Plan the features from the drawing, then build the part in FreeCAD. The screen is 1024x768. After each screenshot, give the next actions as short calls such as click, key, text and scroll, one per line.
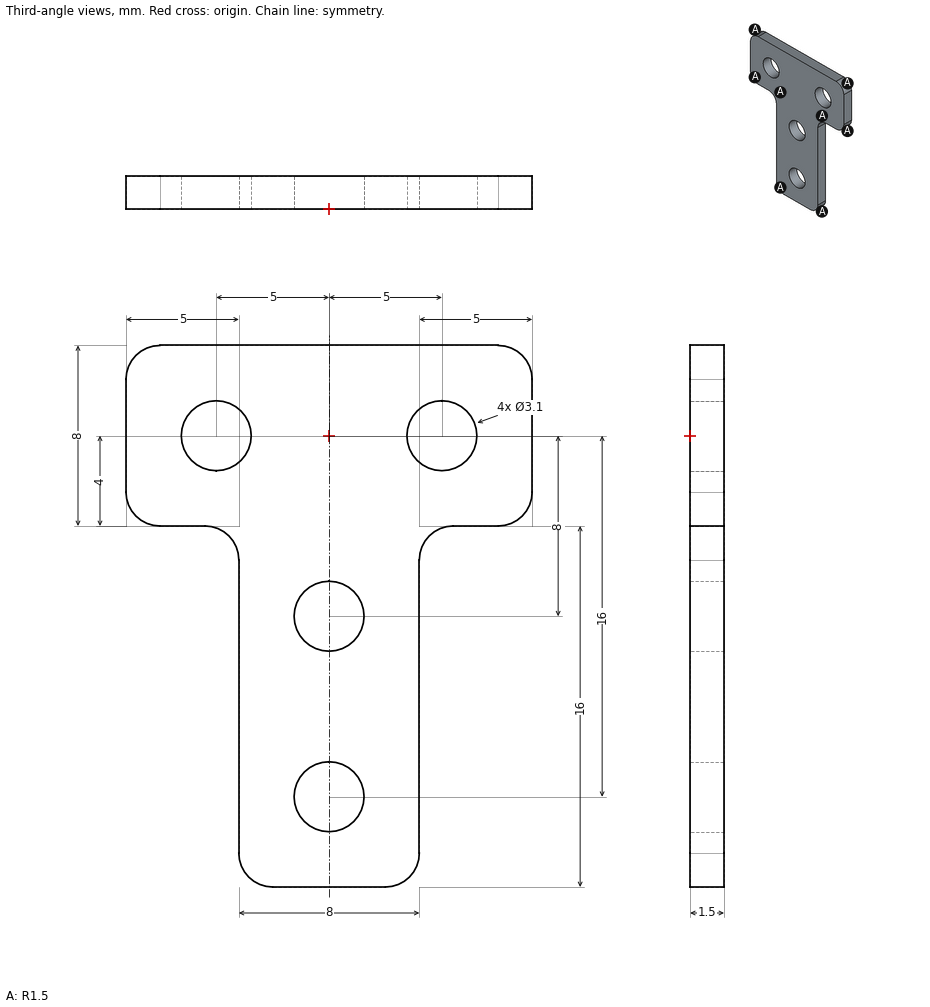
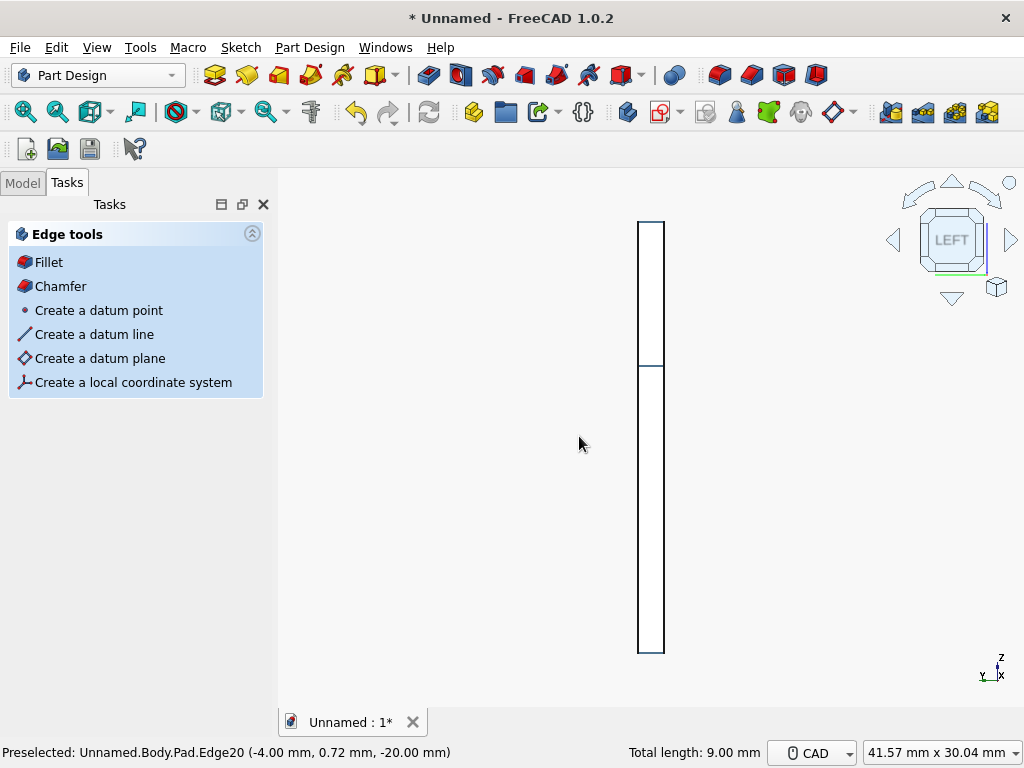
key(v)
key(3)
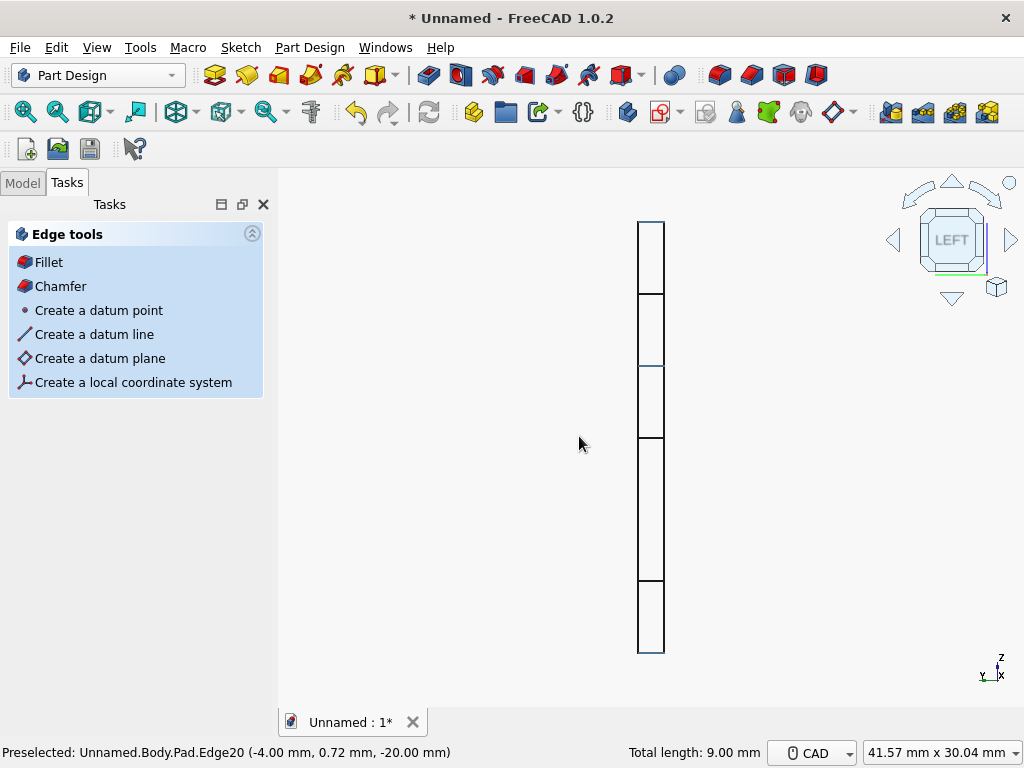
key(0)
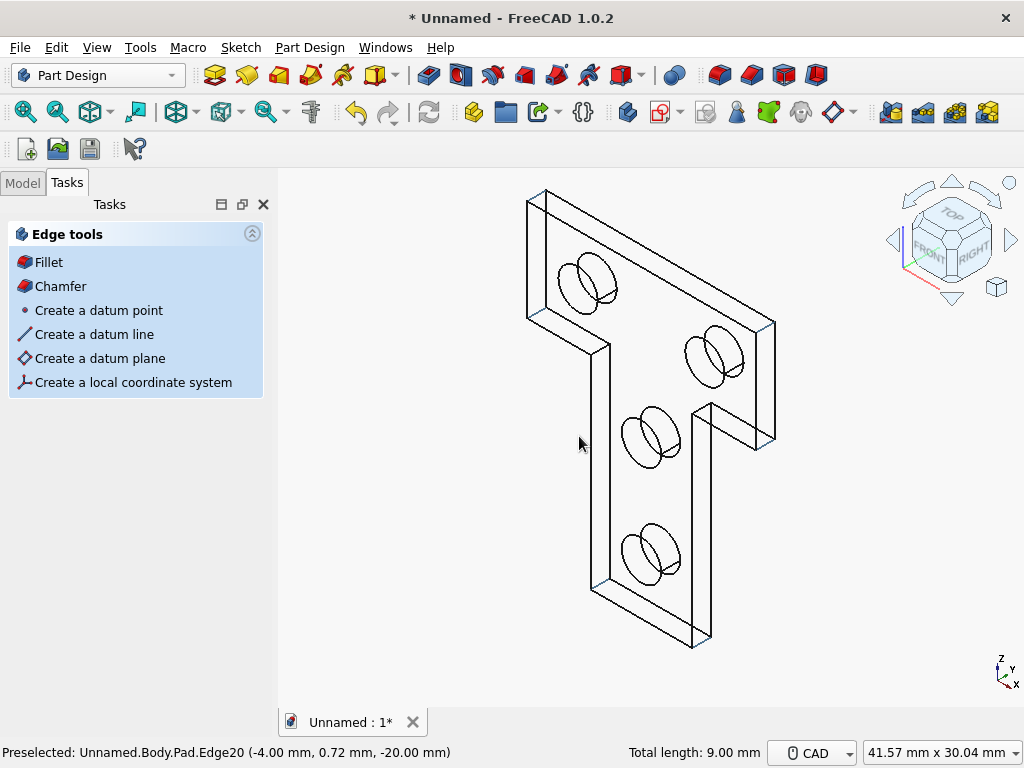
click(702, 407, ctrl)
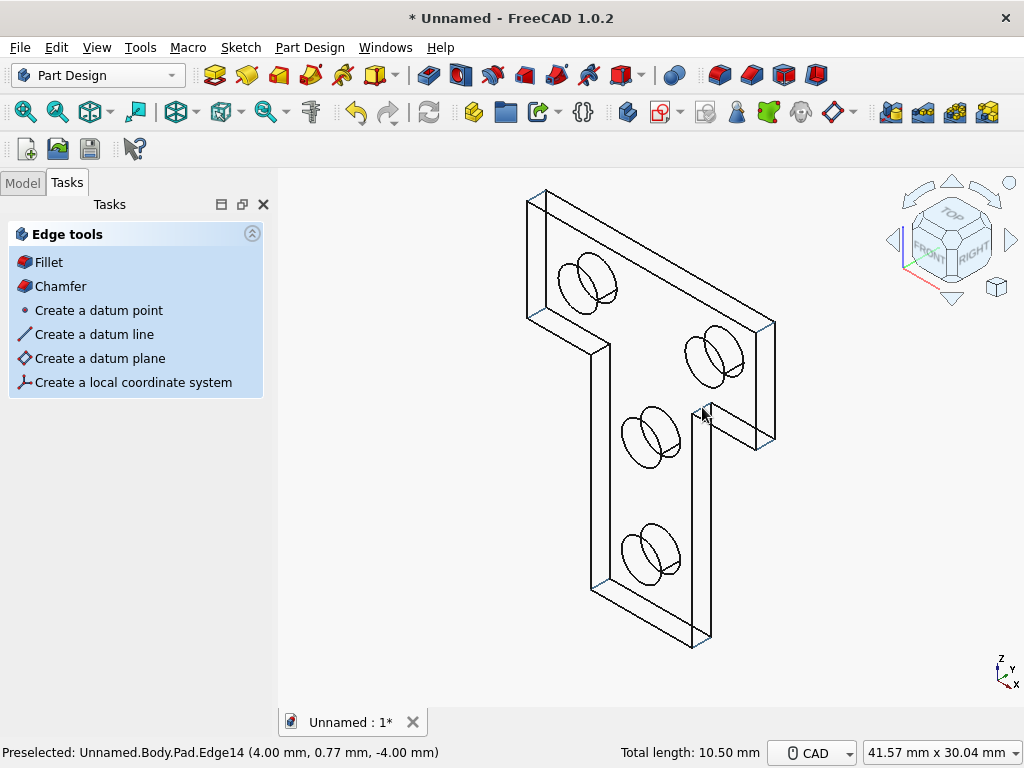
click(600, 349, ctrl)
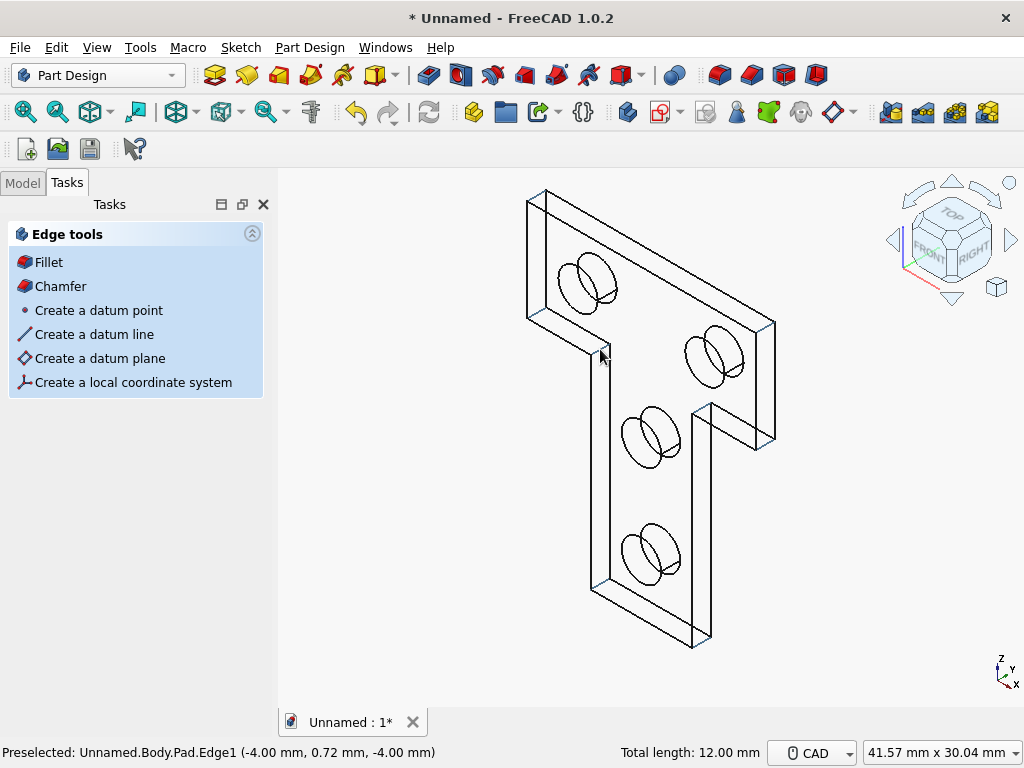
key(v)
key(1)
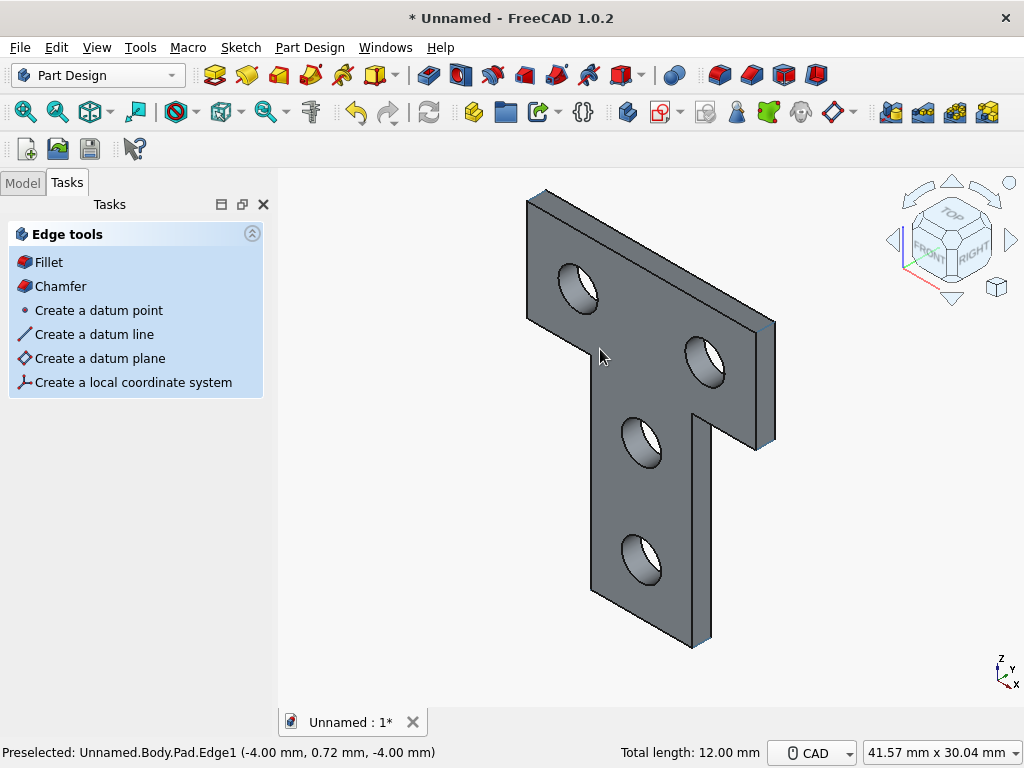
click(720, 76)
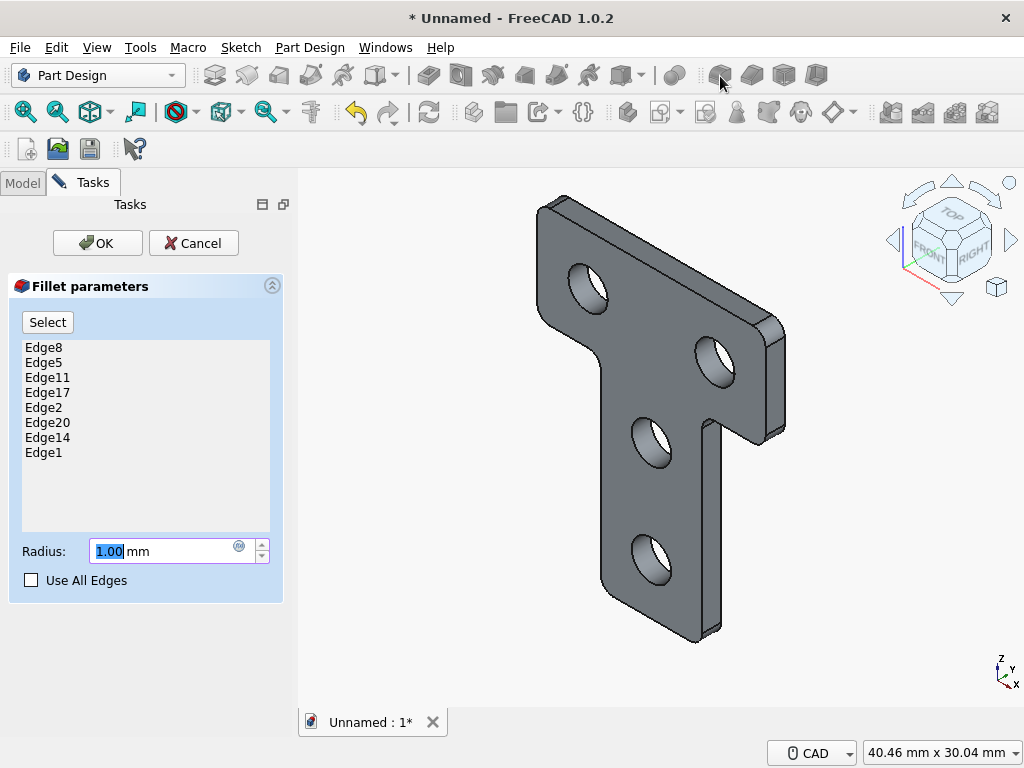
text(1.5)
key(Tab)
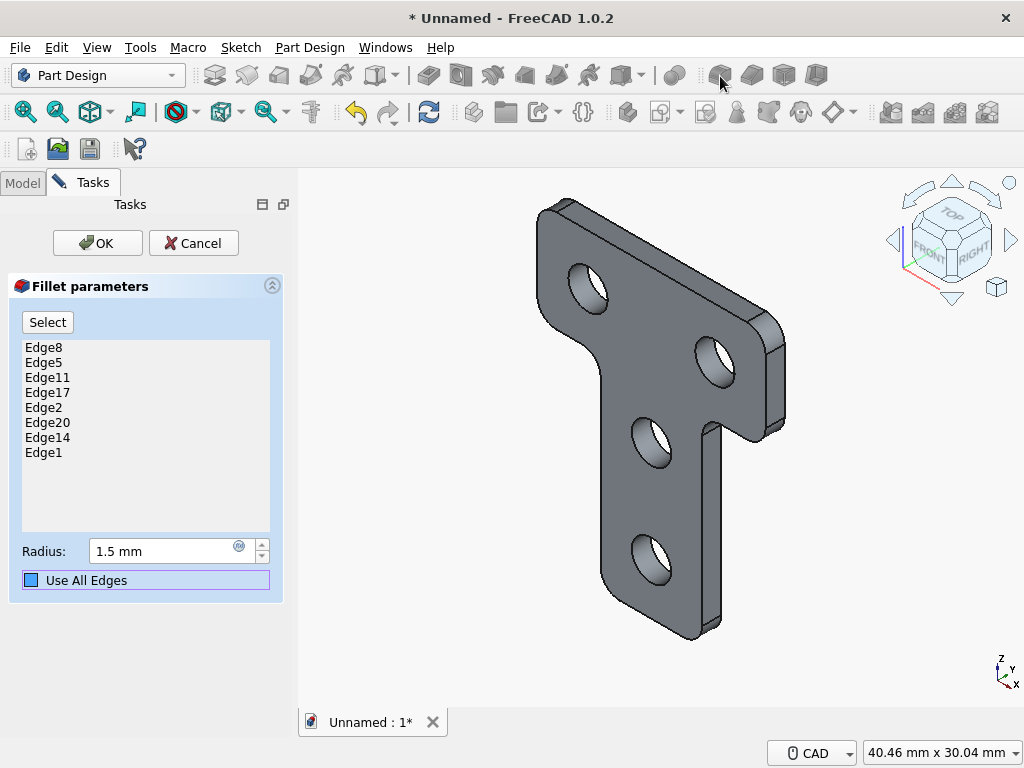
click(98, 243)